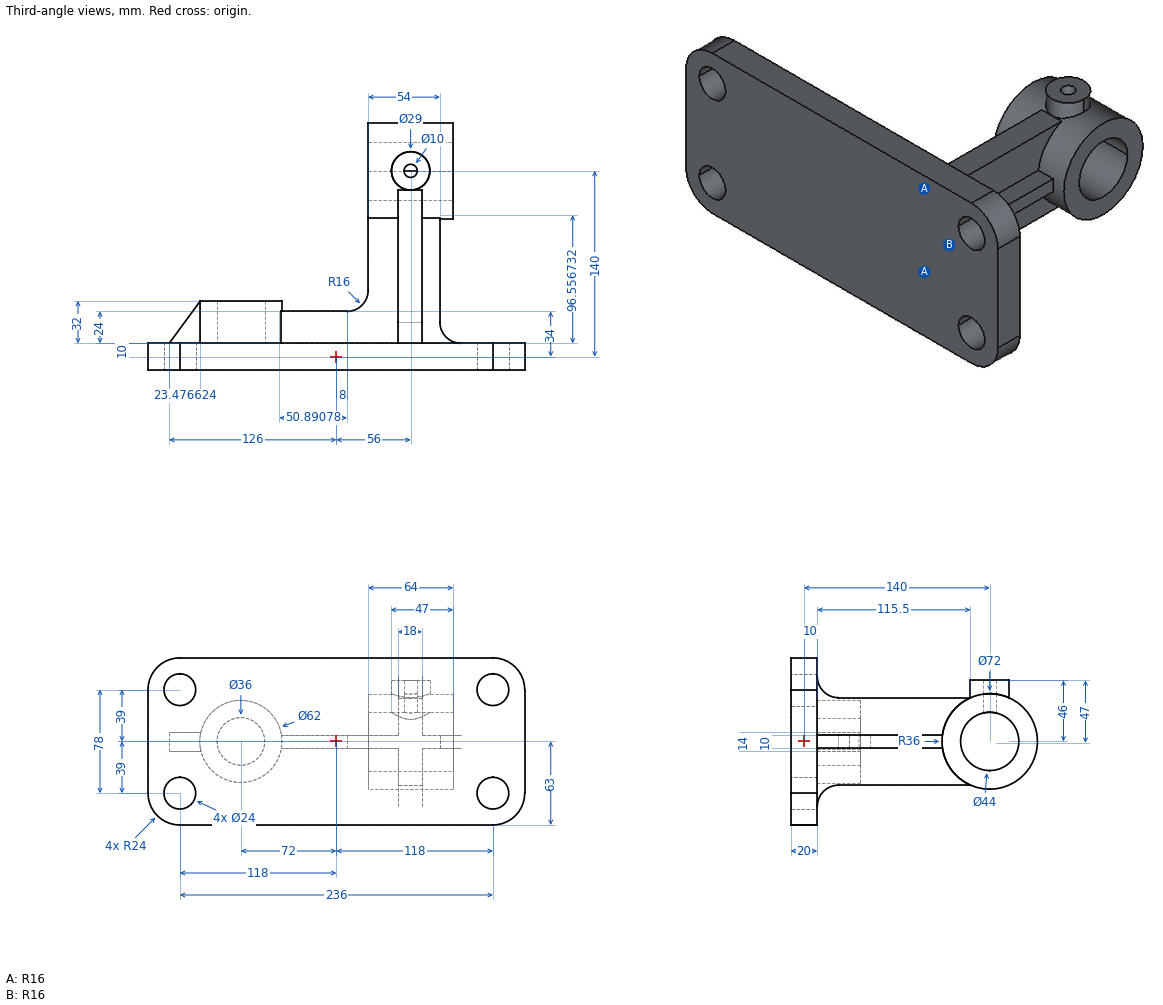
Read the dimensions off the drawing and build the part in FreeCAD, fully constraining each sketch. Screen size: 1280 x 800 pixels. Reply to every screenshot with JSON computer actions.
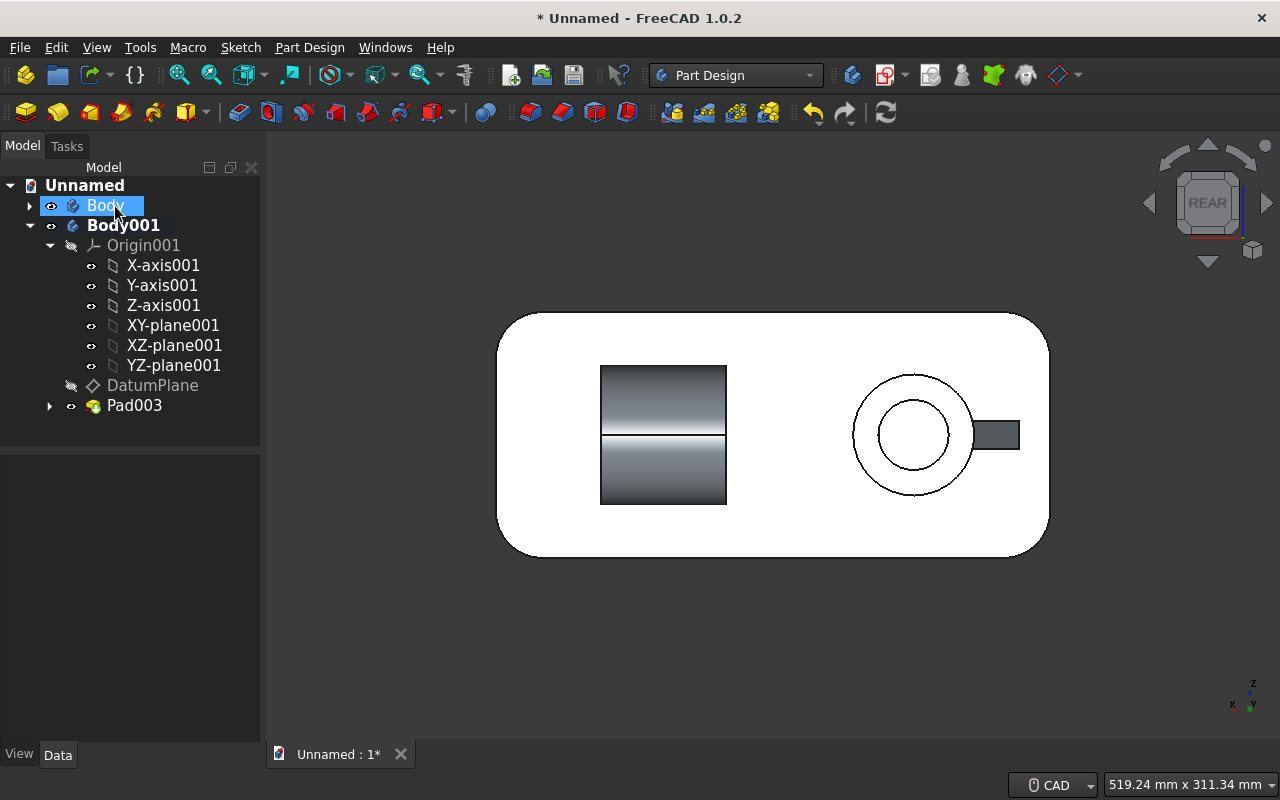
{"action": "left_click", "coordinate": [180, 76]}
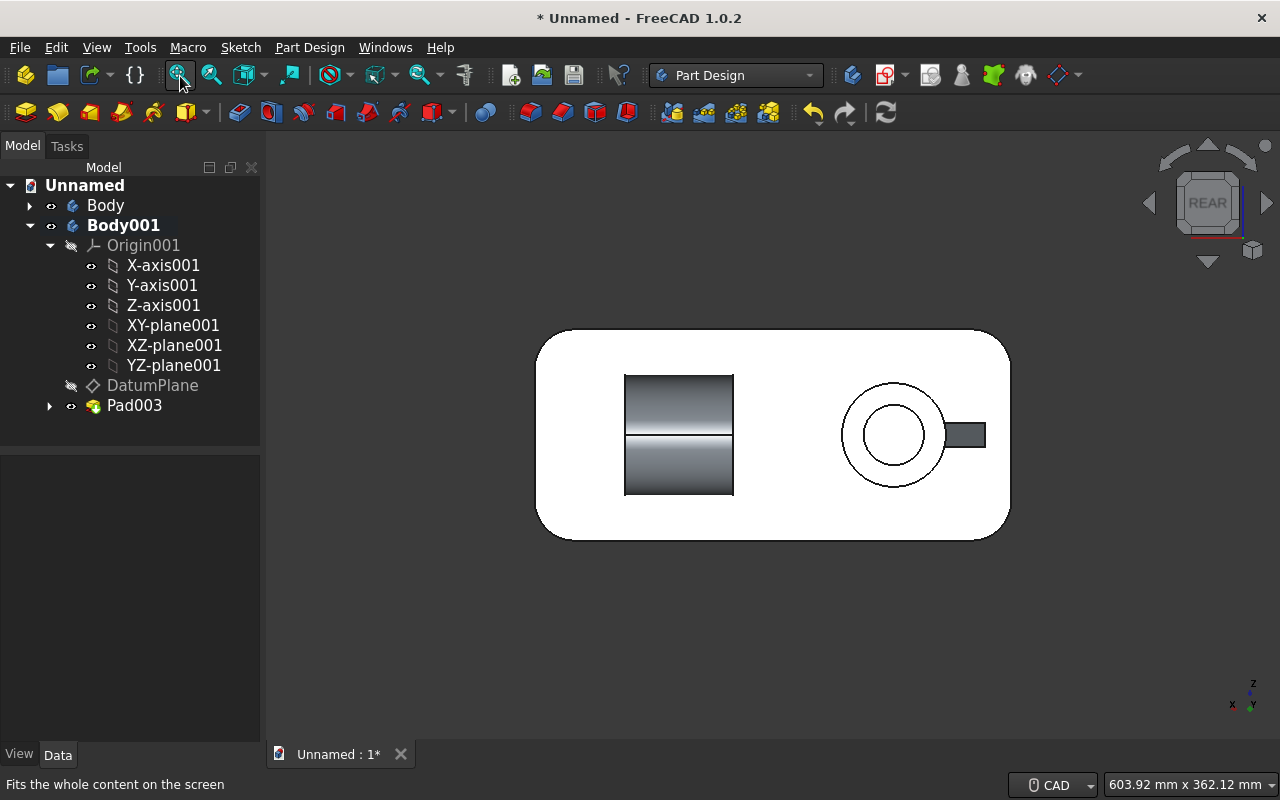
{"action": "double_click", "coordinate": [96, 206]}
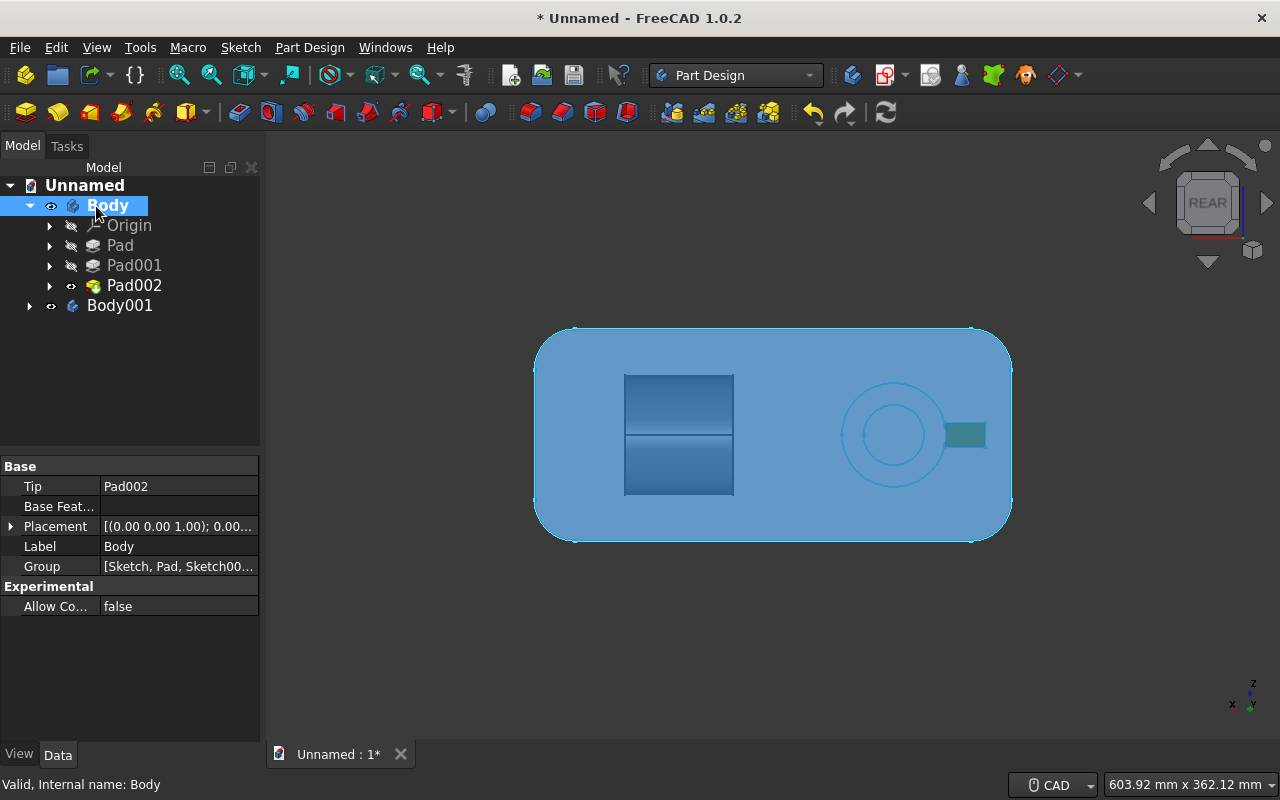
{"action": "left_click", "coordinate": [96, 206]}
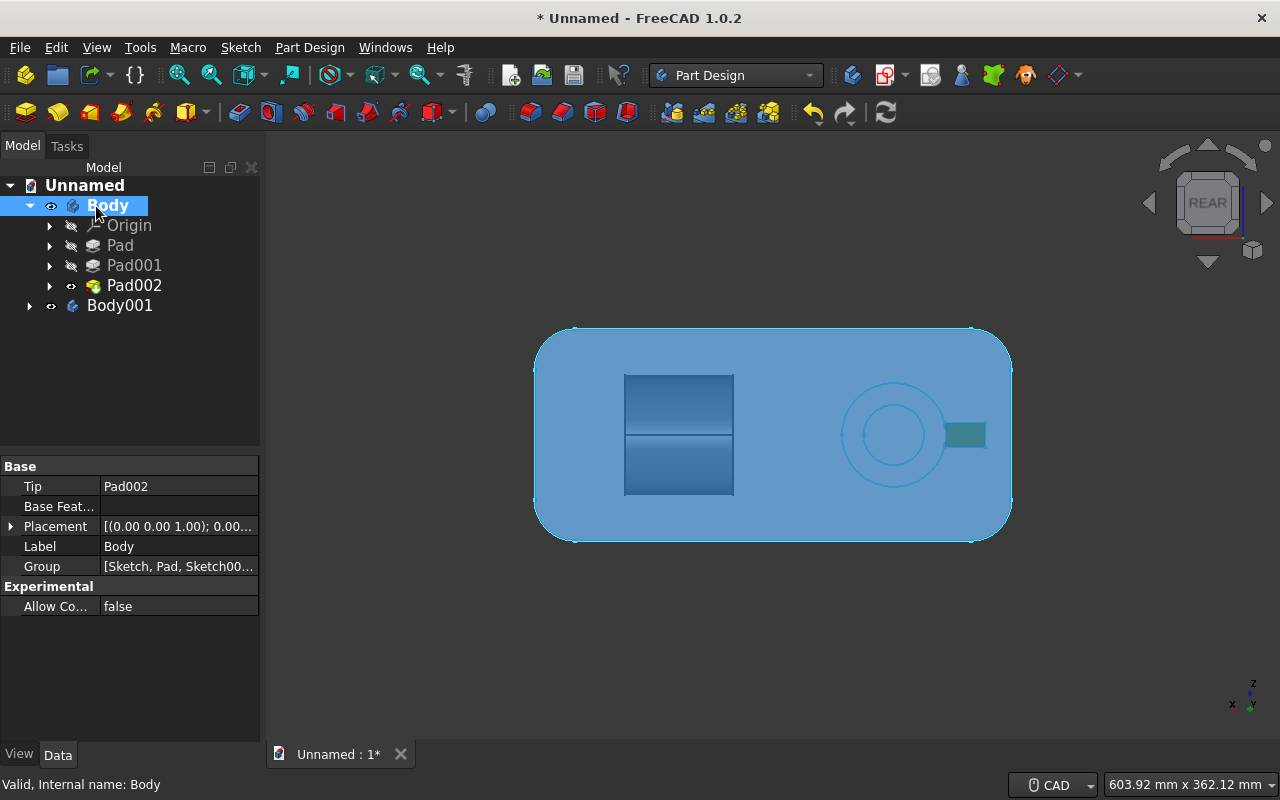
{"action": "left_click", "coordinate": [146, 606]}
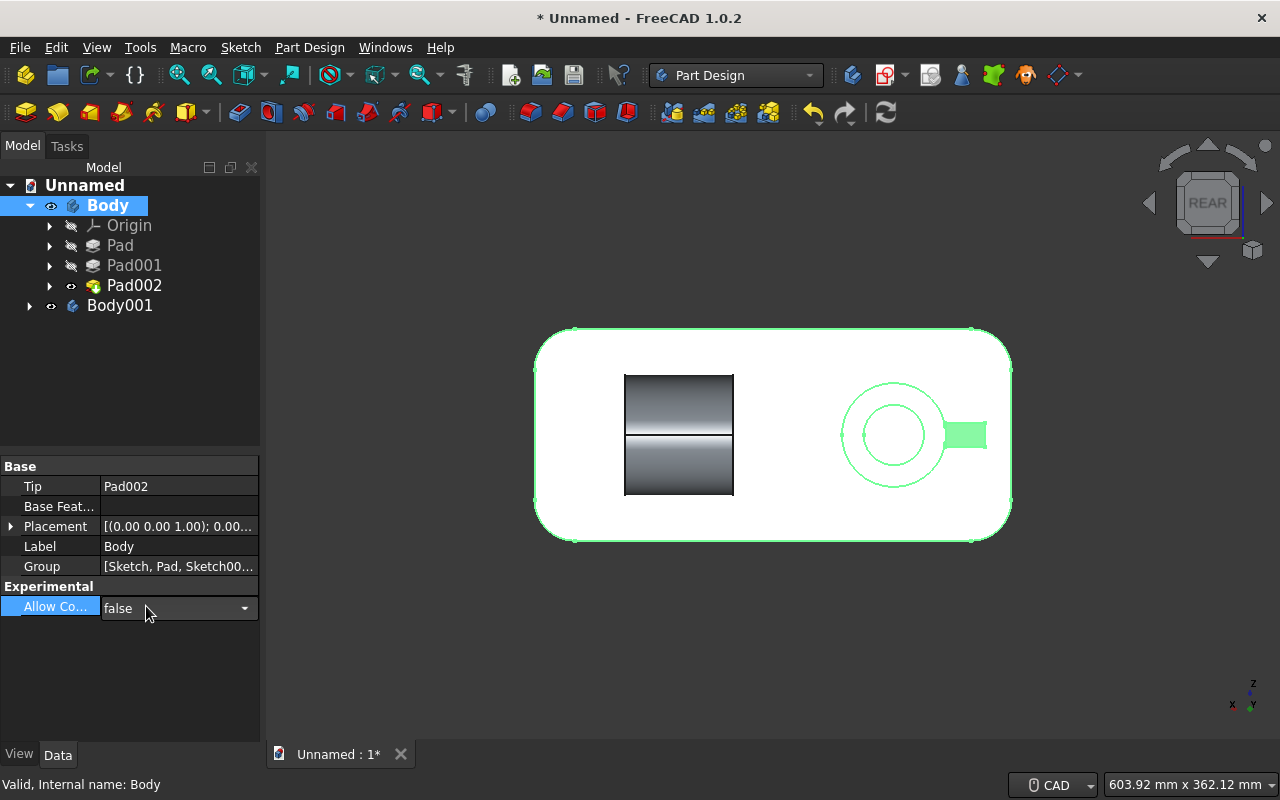
{"action": "left_click", "coordinate": [146, 606]}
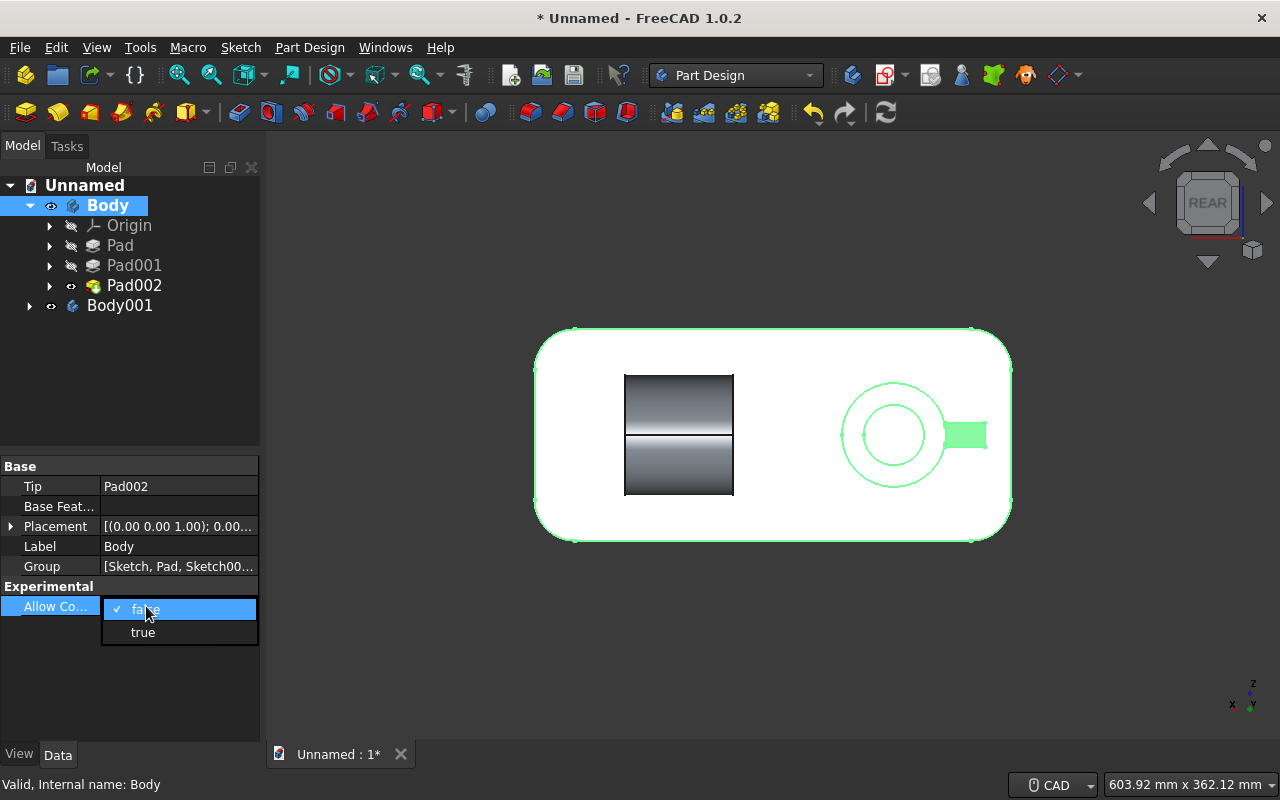
{"action": "left_click", "coordinate": [179, 632]}
{"action": "key", "text": "Return"}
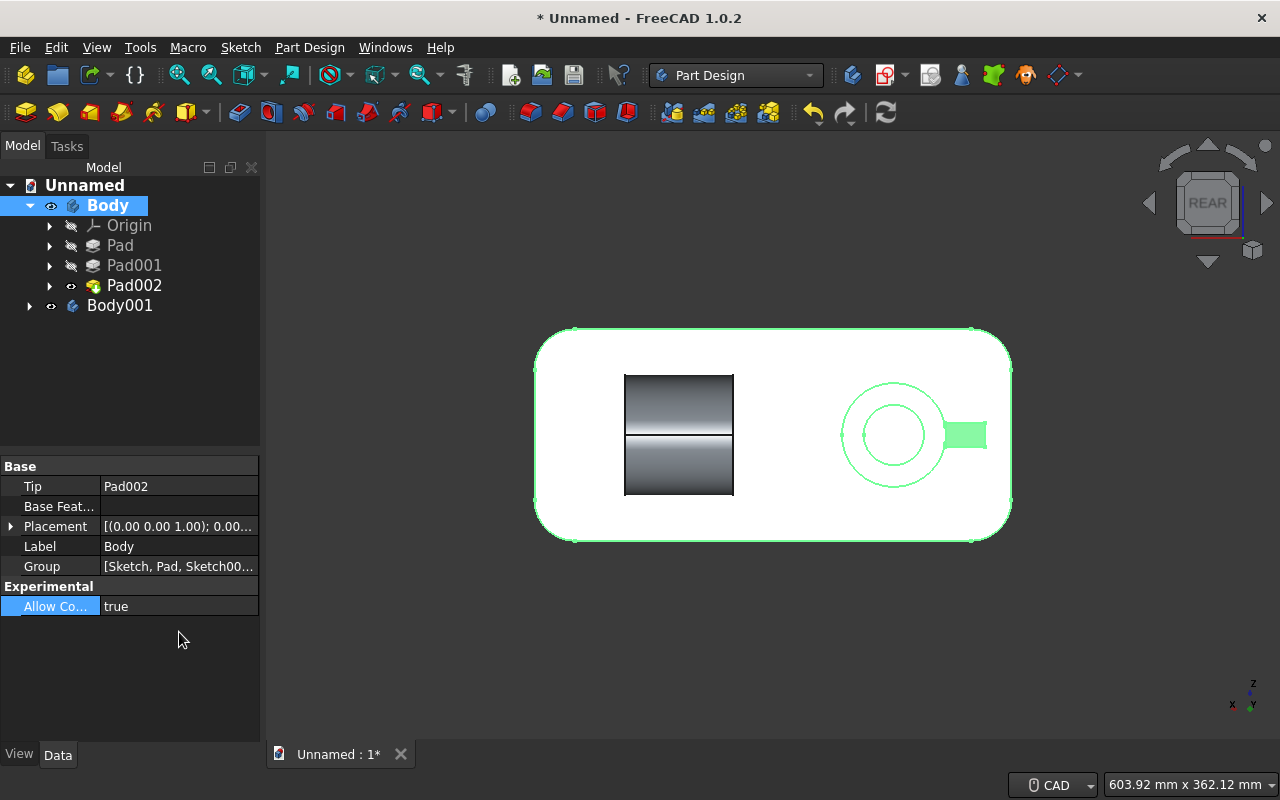
{"action": "left_click", "coordinate": [96, 306]}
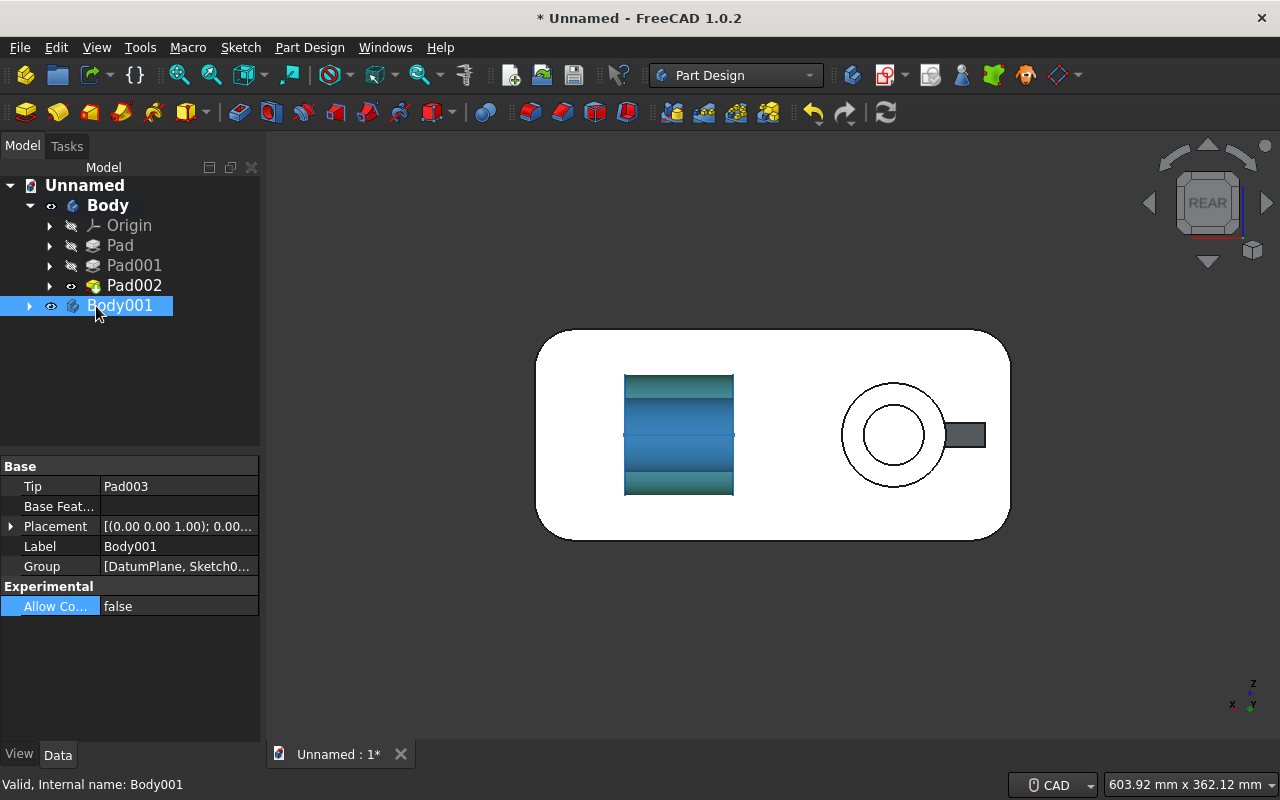
{"action": "left_click", "coordinate": [486, 112]}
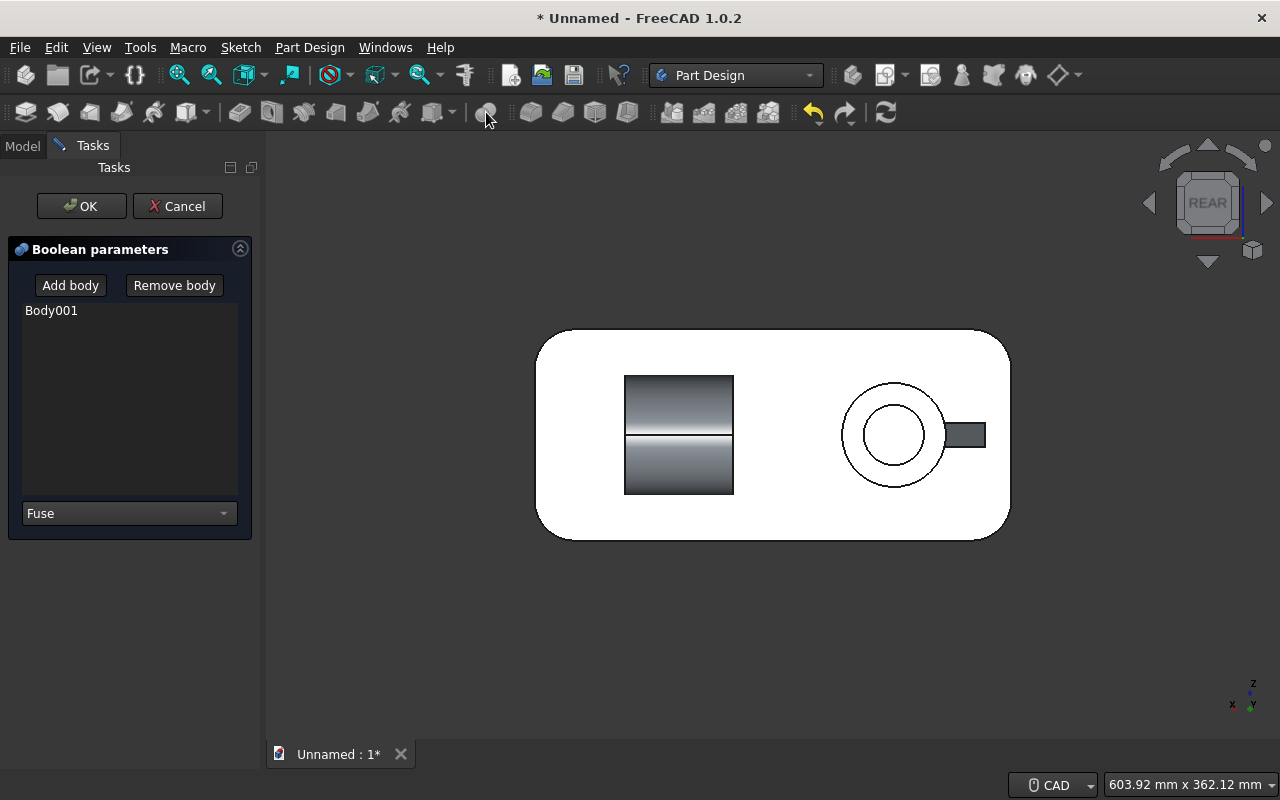
{"action": "left_click", "coordinate": [82, 206]}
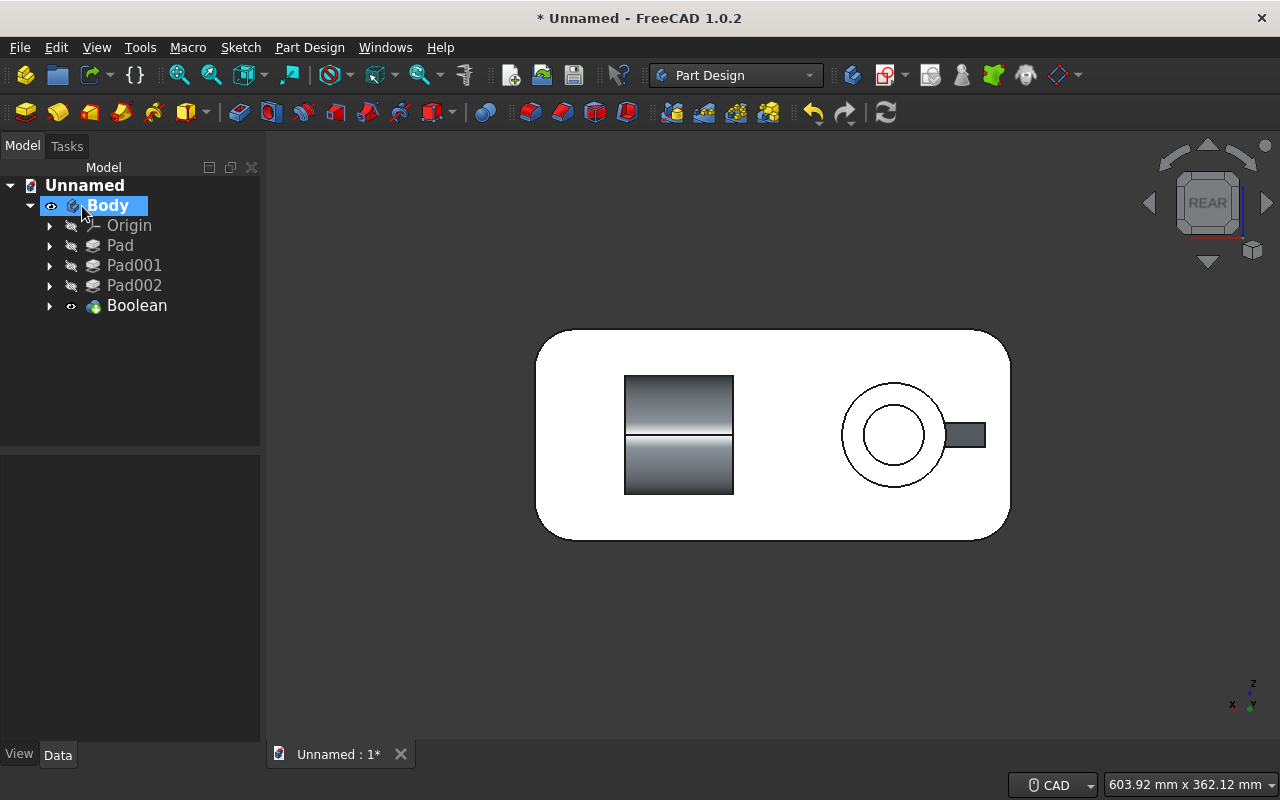
{"action": "left_click", "coordinate": [886, 76]}